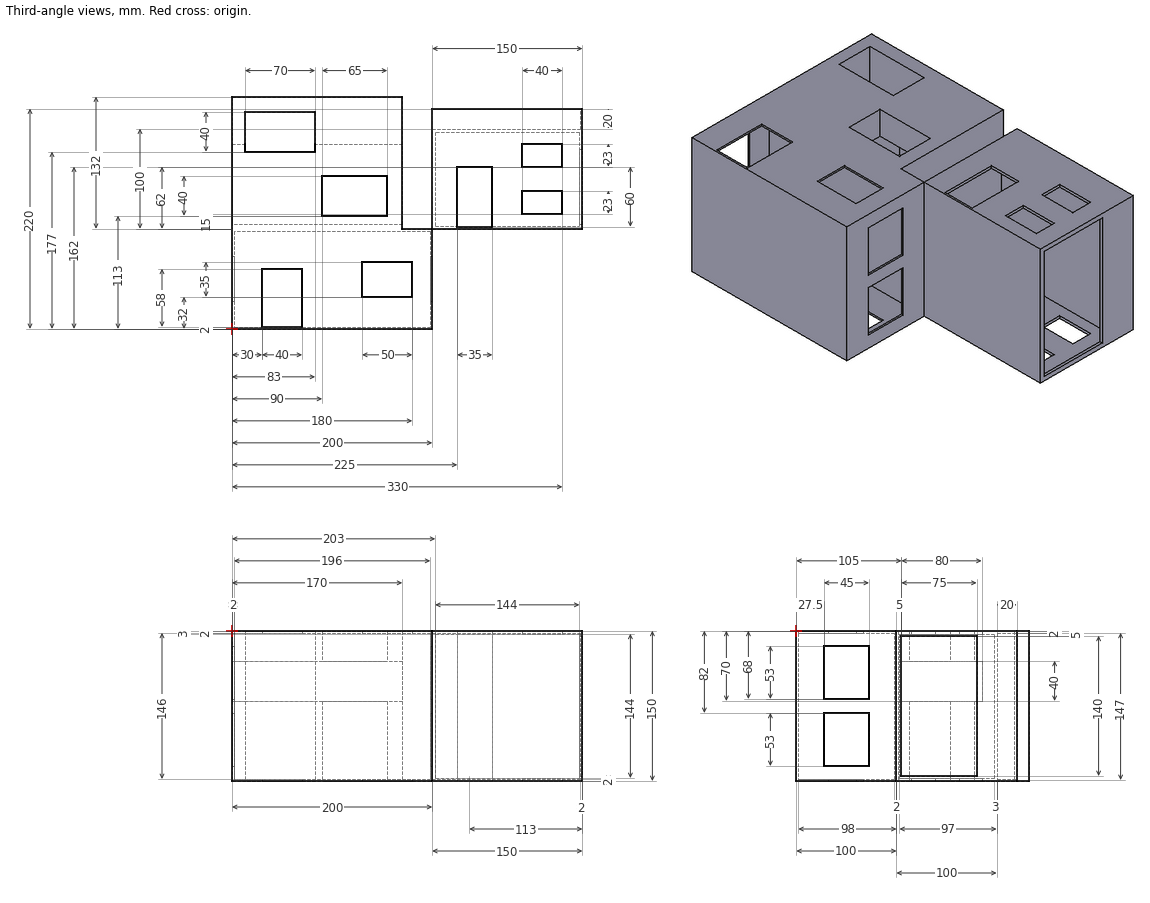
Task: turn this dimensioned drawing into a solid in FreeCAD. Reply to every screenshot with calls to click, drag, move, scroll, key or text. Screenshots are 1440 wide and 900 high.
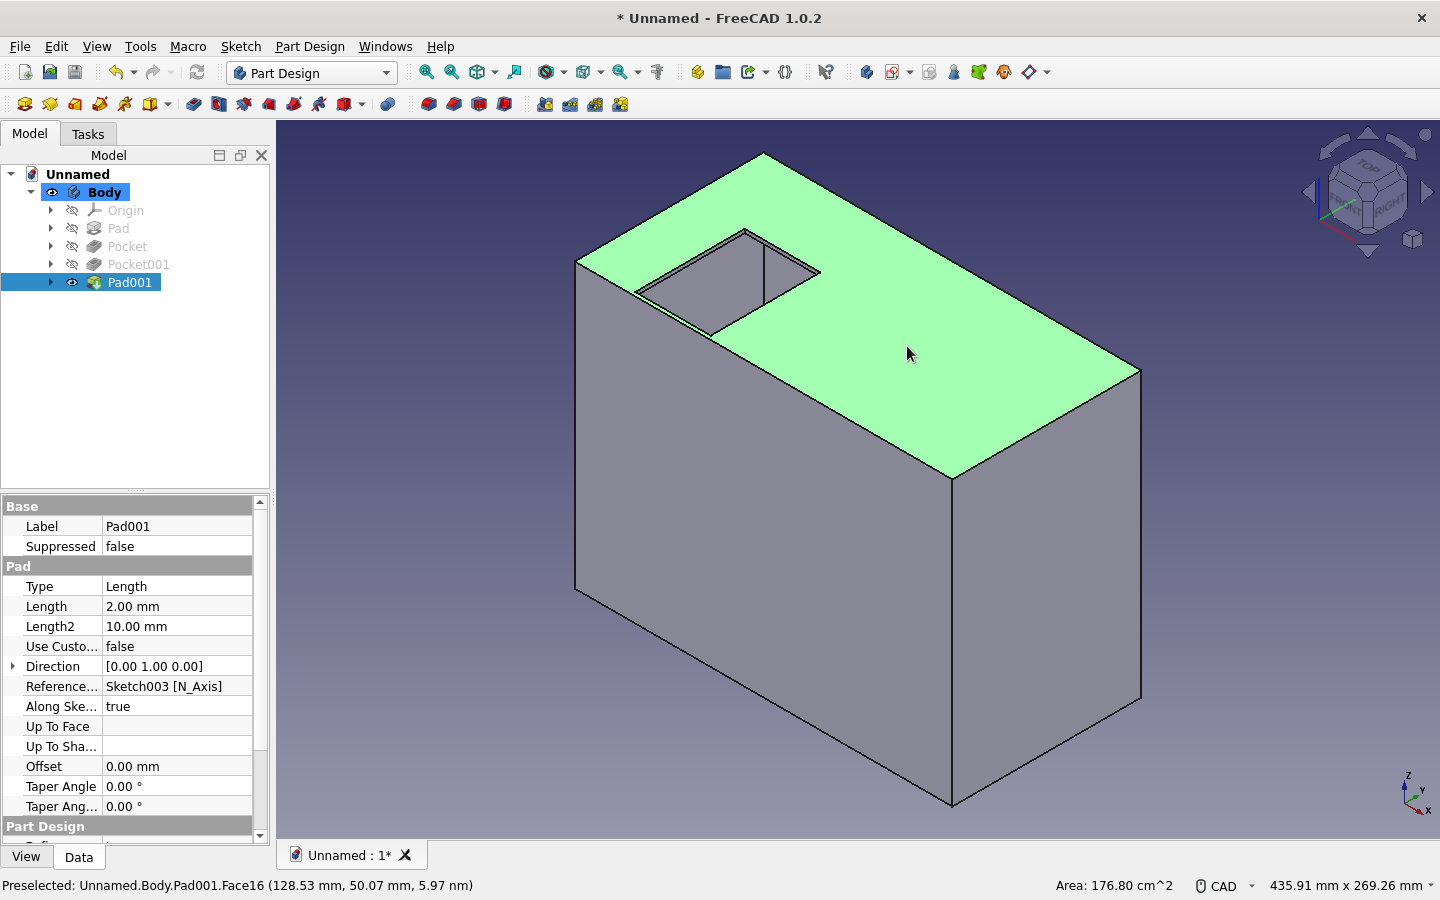
click(892, 72)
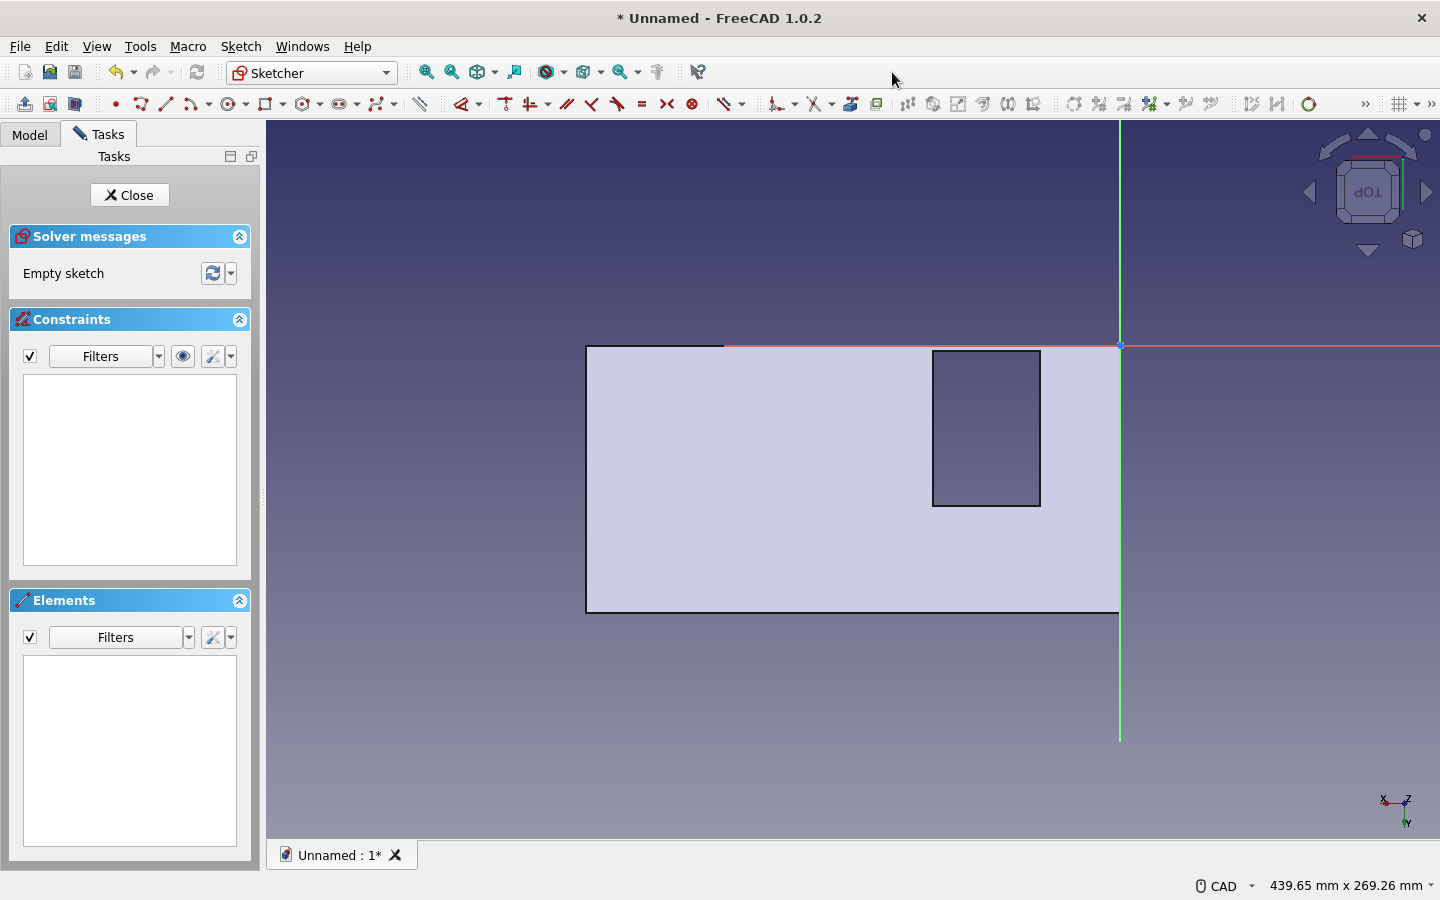
scroll(686, 478, up, 8)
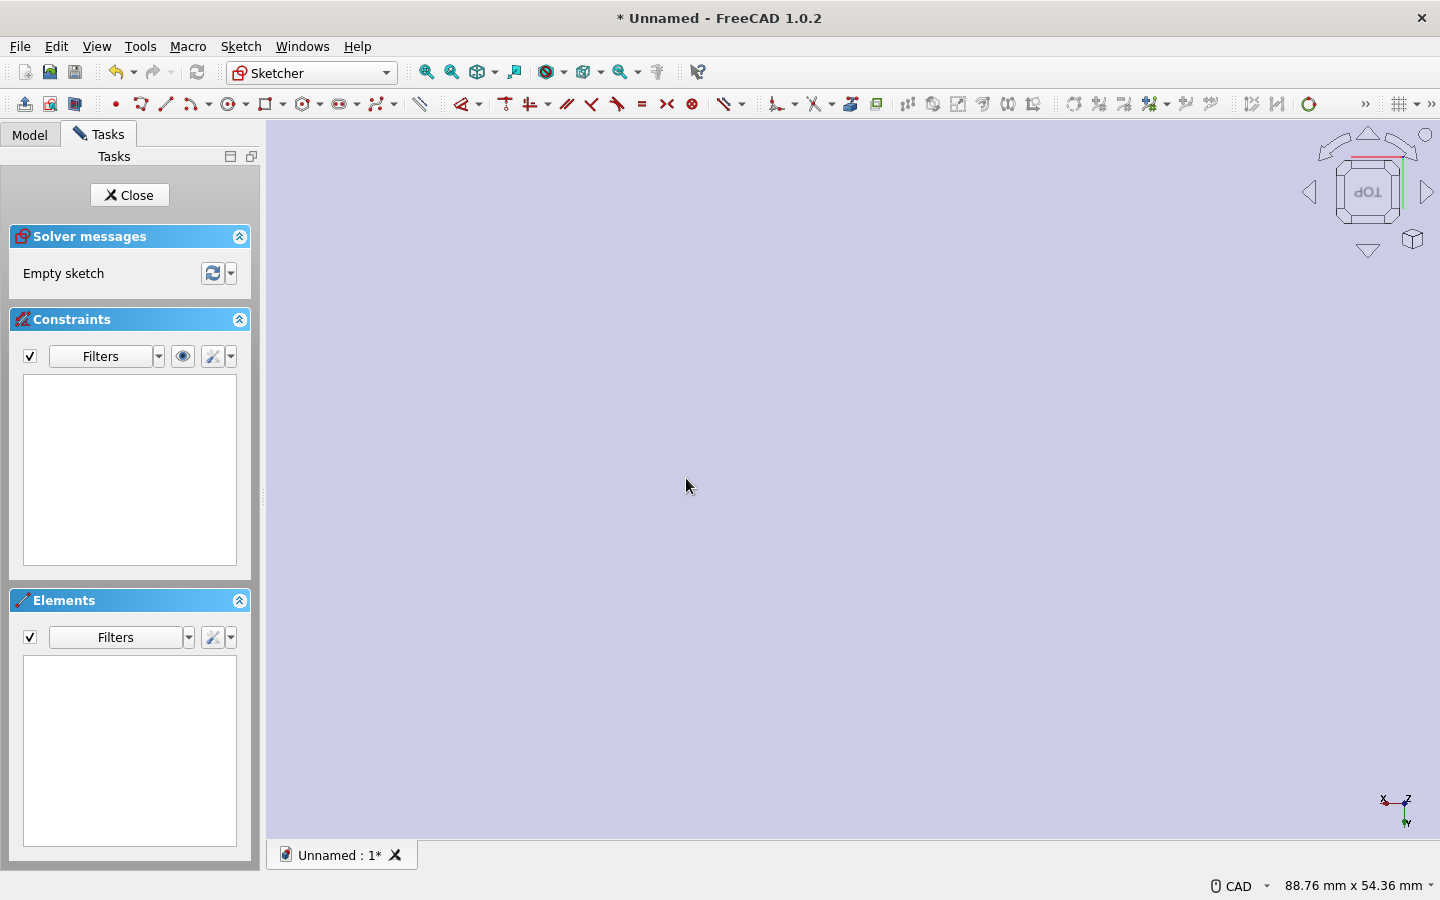
click(264, 104)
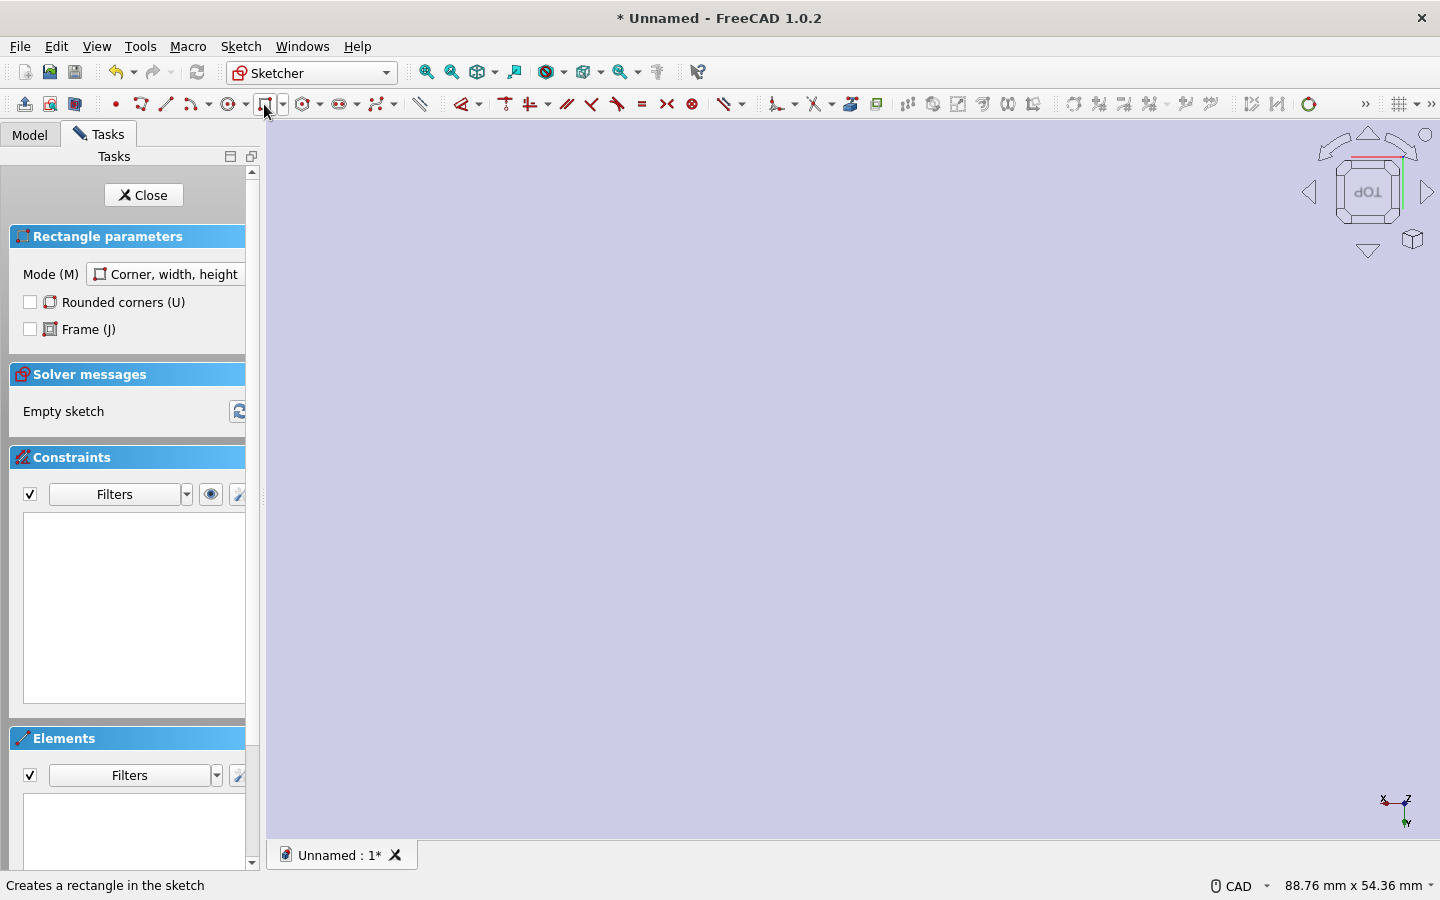
click(454, 245)
move(1115, 708)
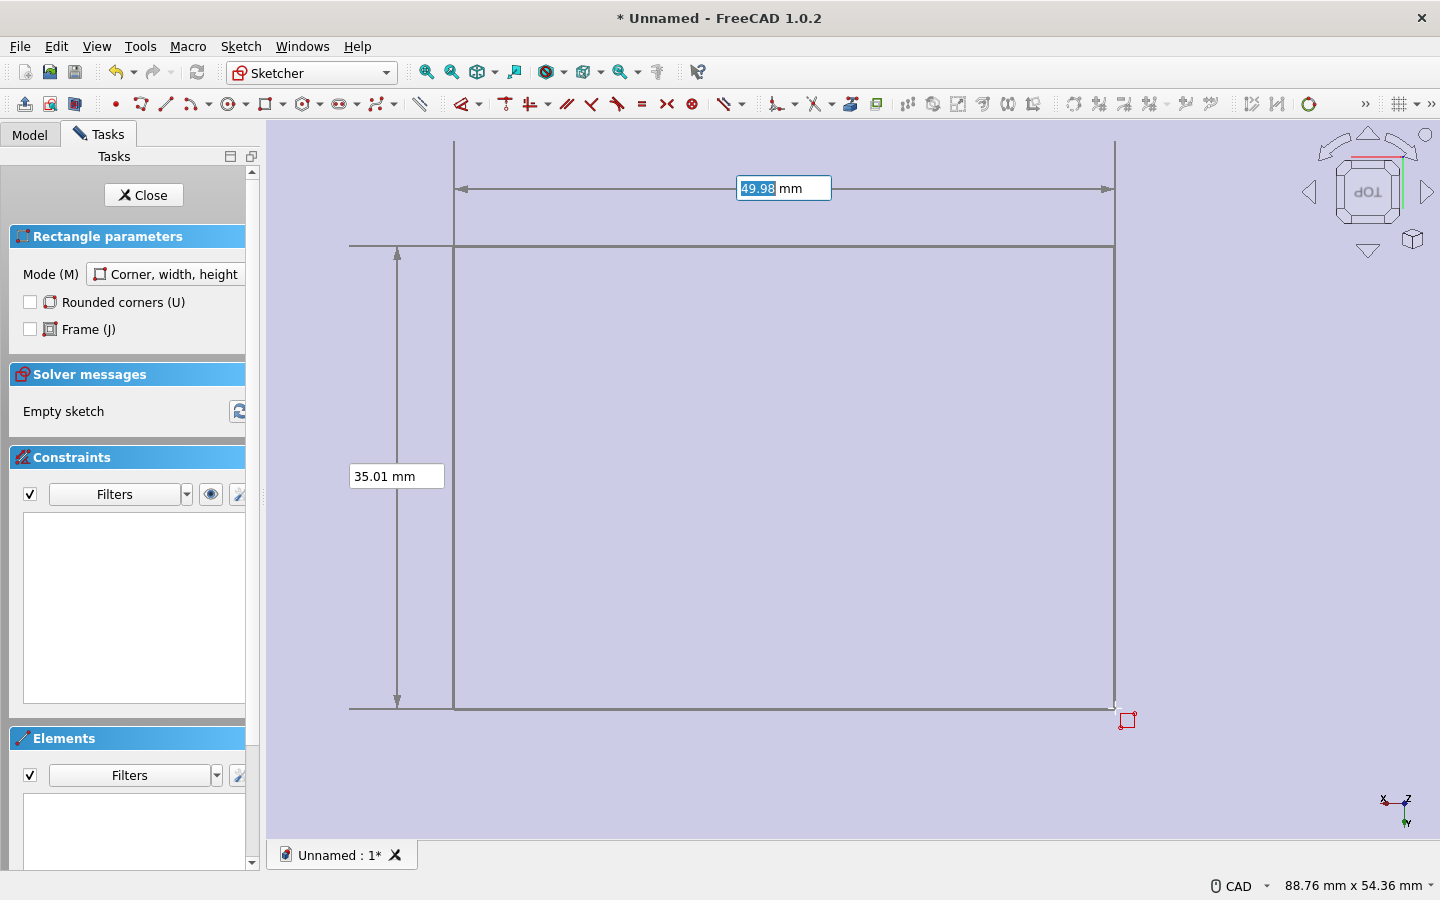
text(50)
key(Tab)
text(35)
key(Return)
key(Escape)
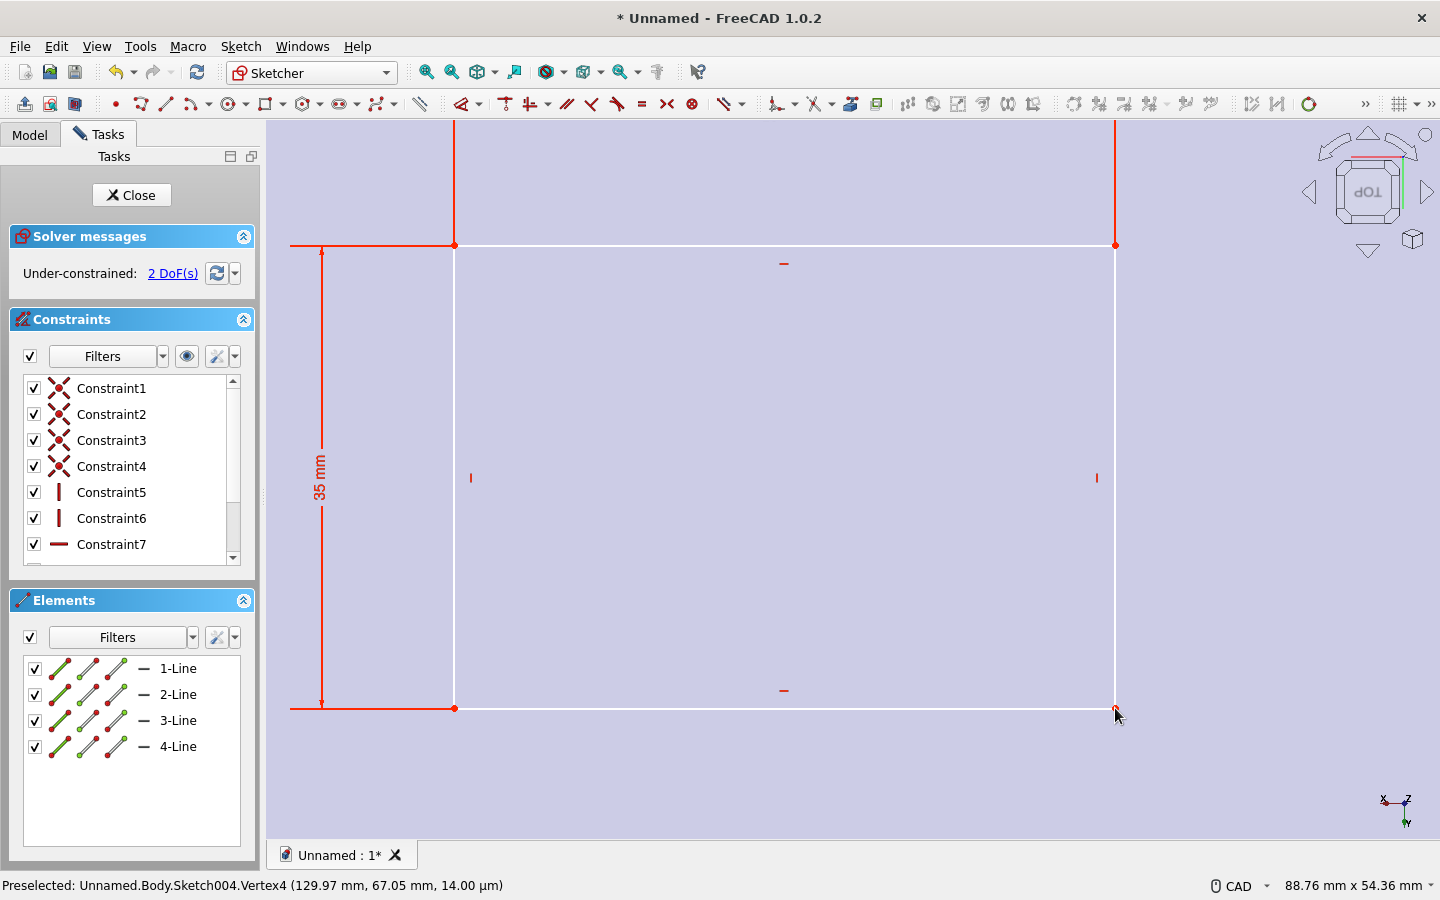
click(460, 104)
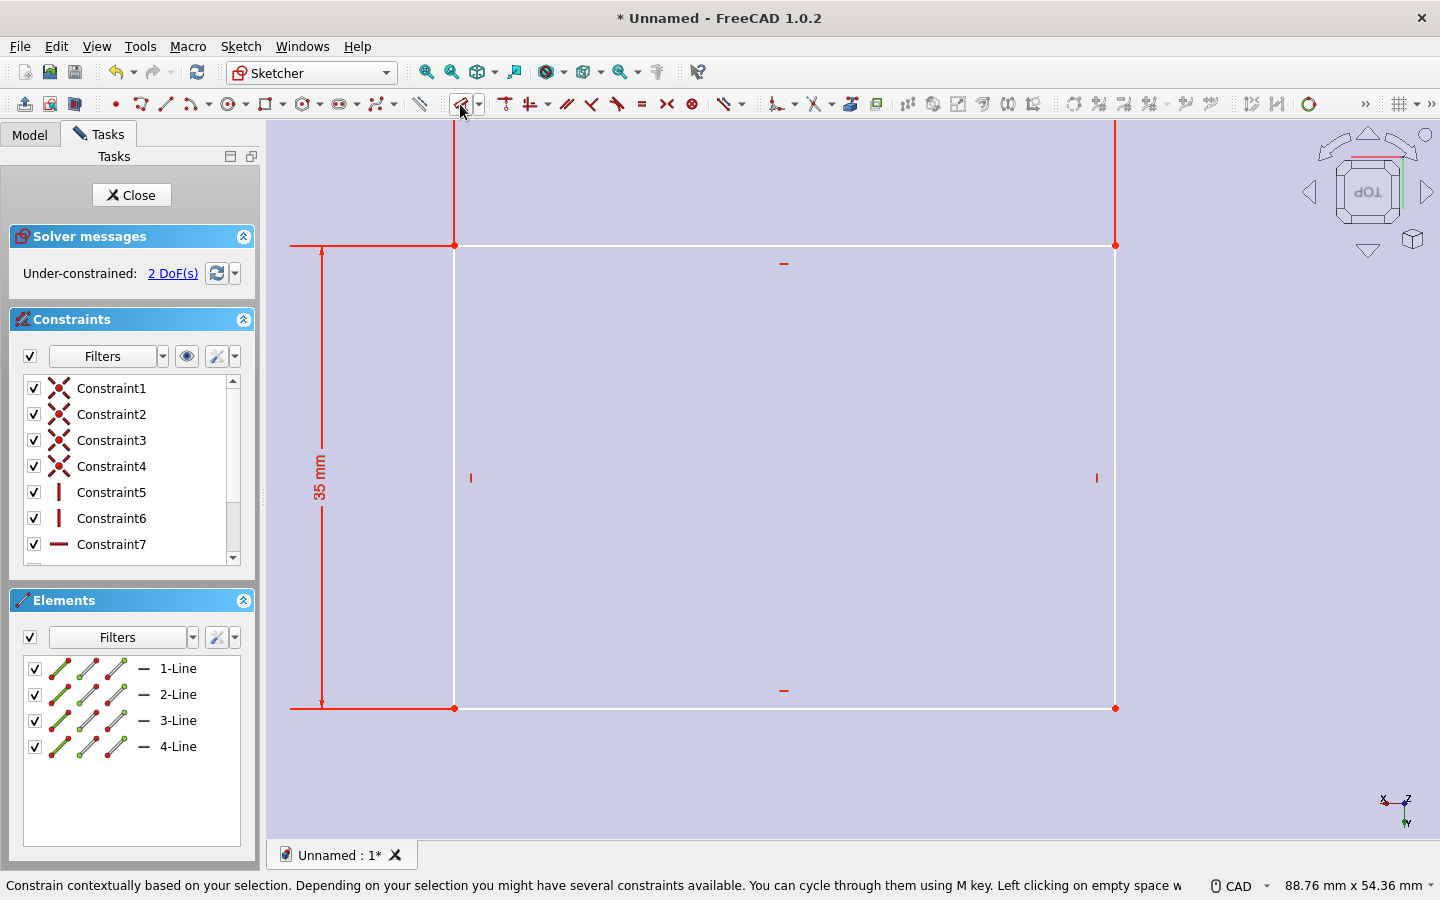
click(454, 246)
click(420, 197)